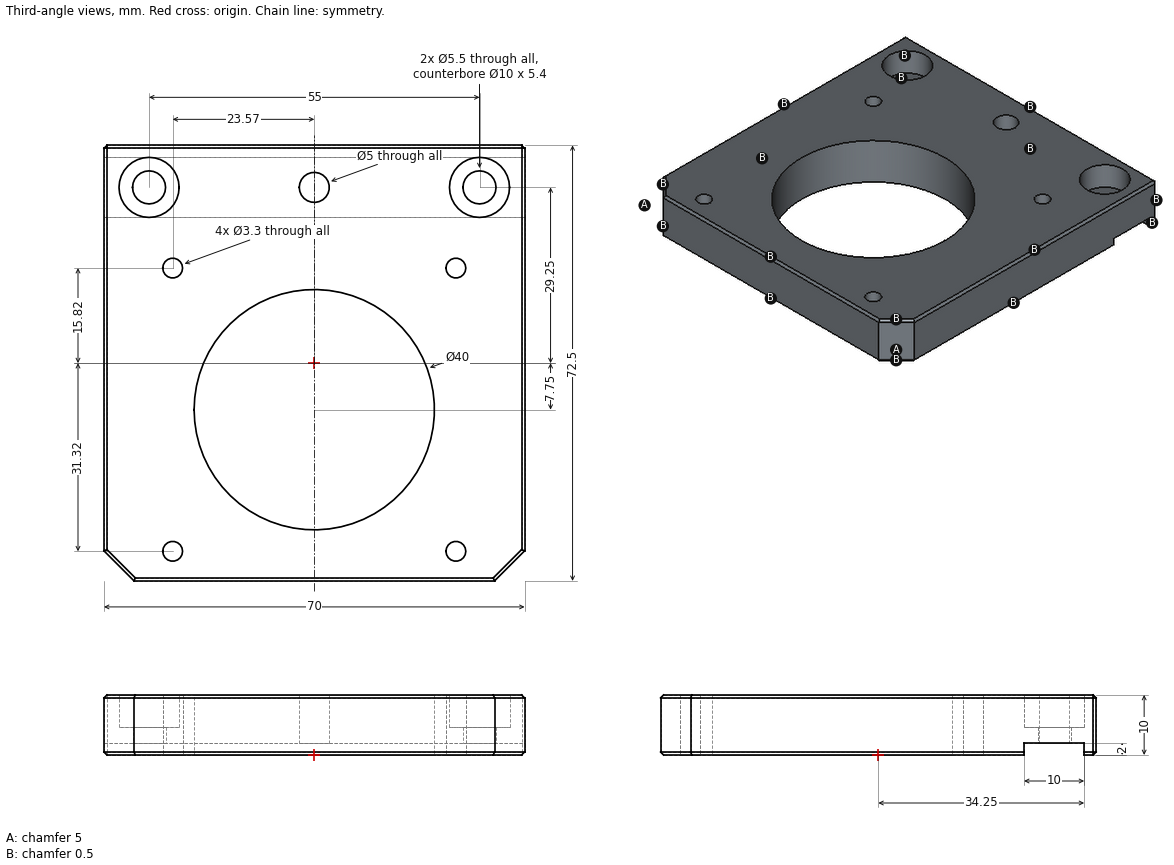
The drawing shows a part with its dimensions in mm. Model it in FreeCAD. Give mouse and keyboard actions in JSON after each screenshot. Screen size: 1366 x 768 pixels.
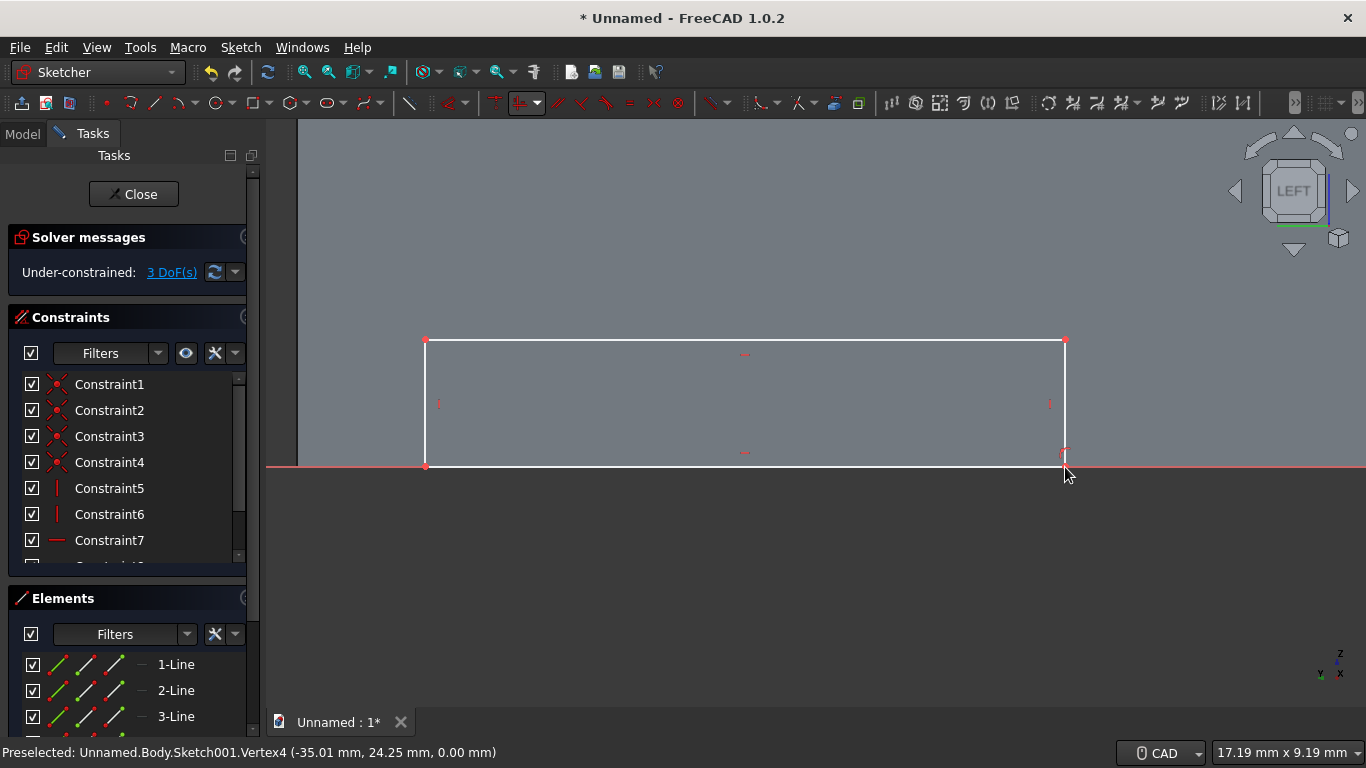
{"action": "left_click", "coordinate": [448, 104]}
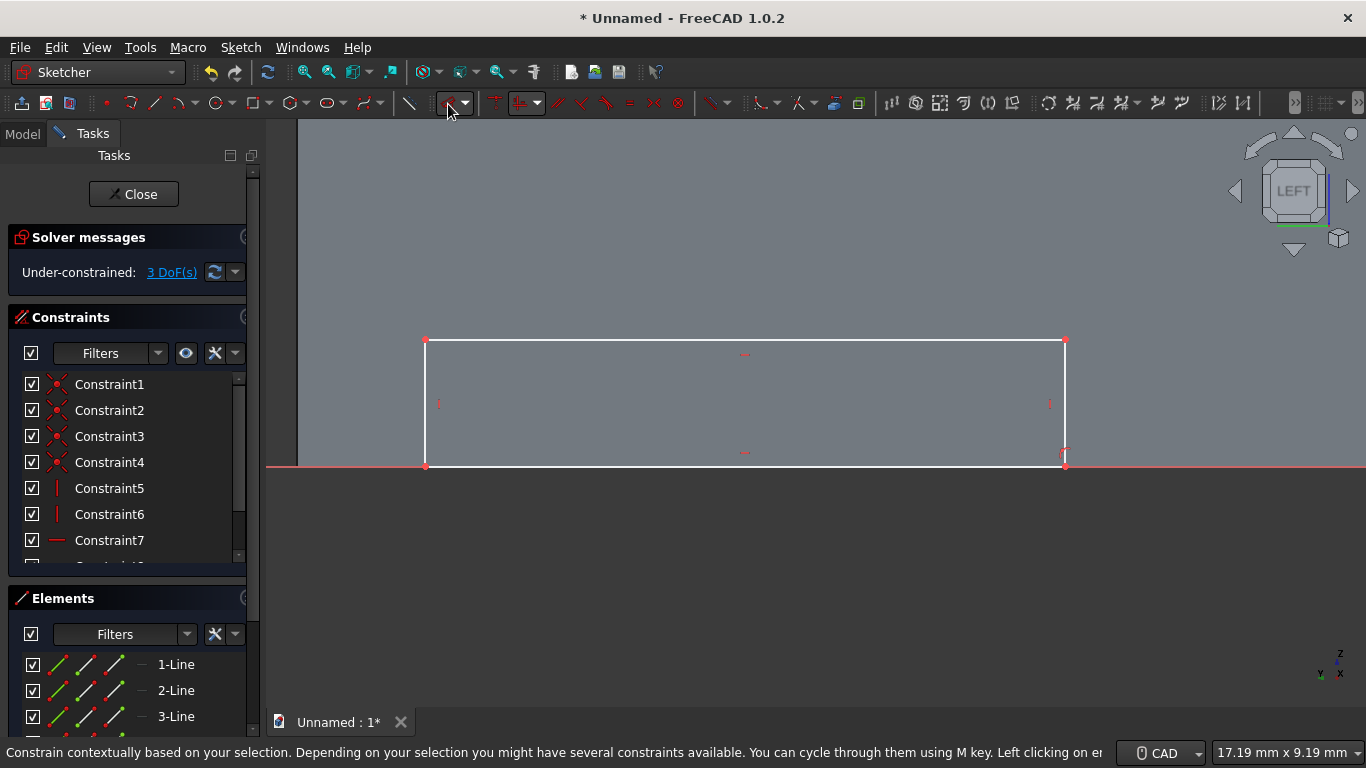
{"action": "left_click", "coordinate": [425, 378]}
{"action": "left_click", "coordinate": [391, 403]}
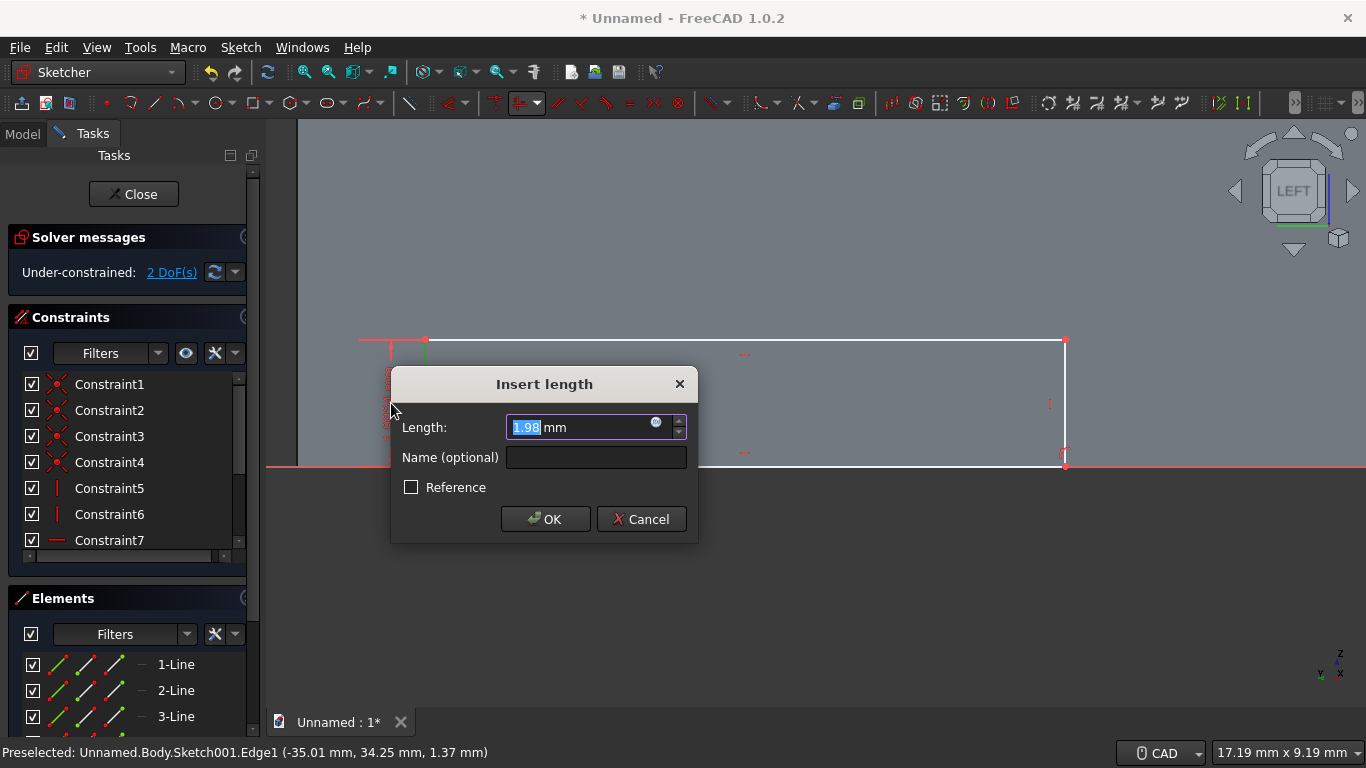
{"action": "type", "text": "2"}
{"action": "key", "text": "Return"}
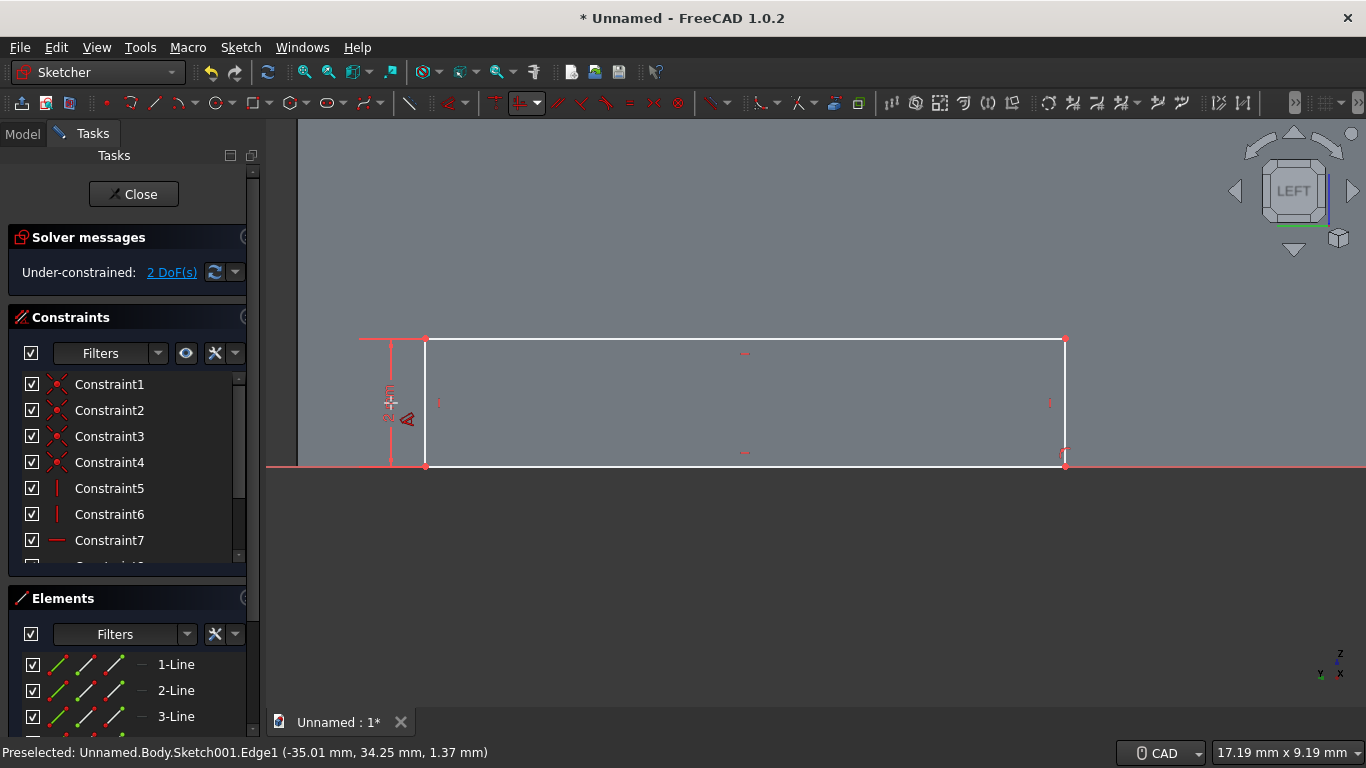
{"action": "left_click", "coordinate": [617, 467]}
{"action": "left_click", "coordinate": [745, 501]}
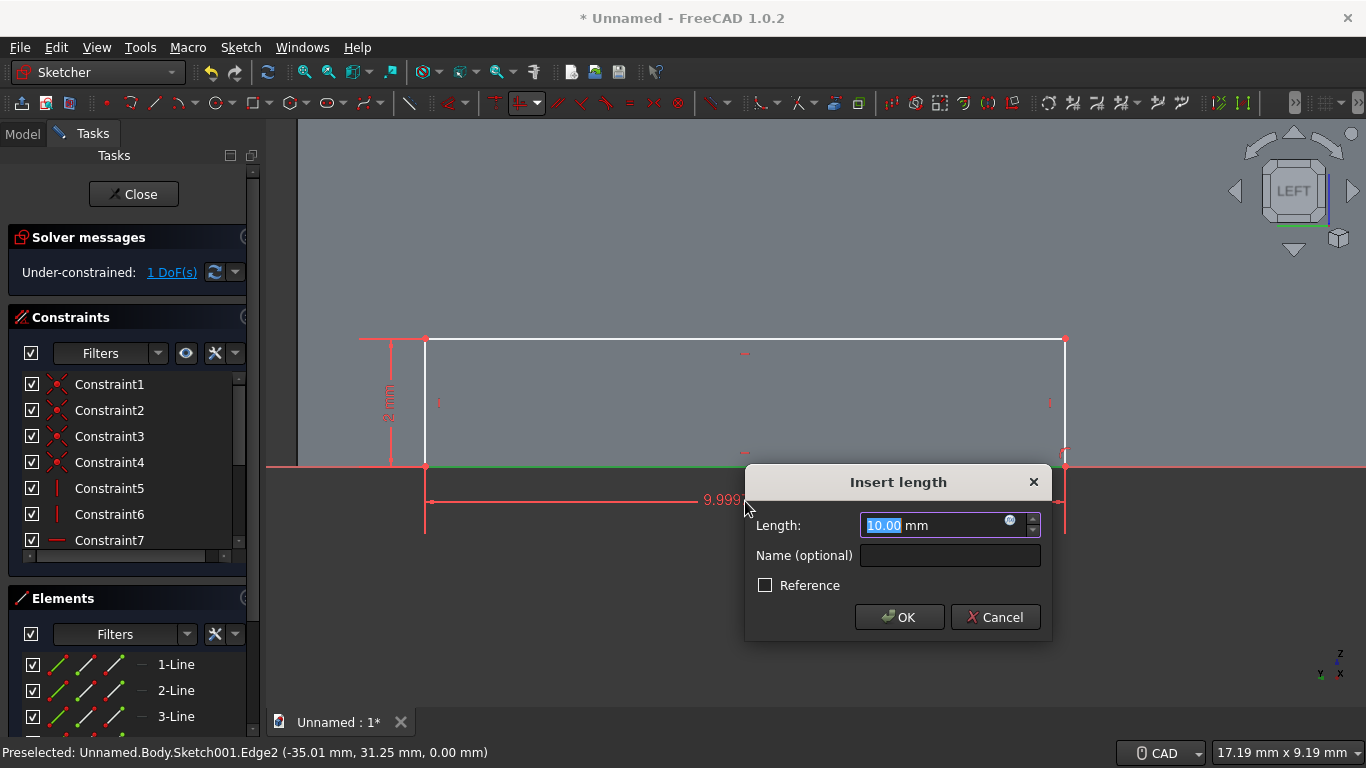
{"action": "type", "text": "10"}
{"action": "key", "text": "Return"}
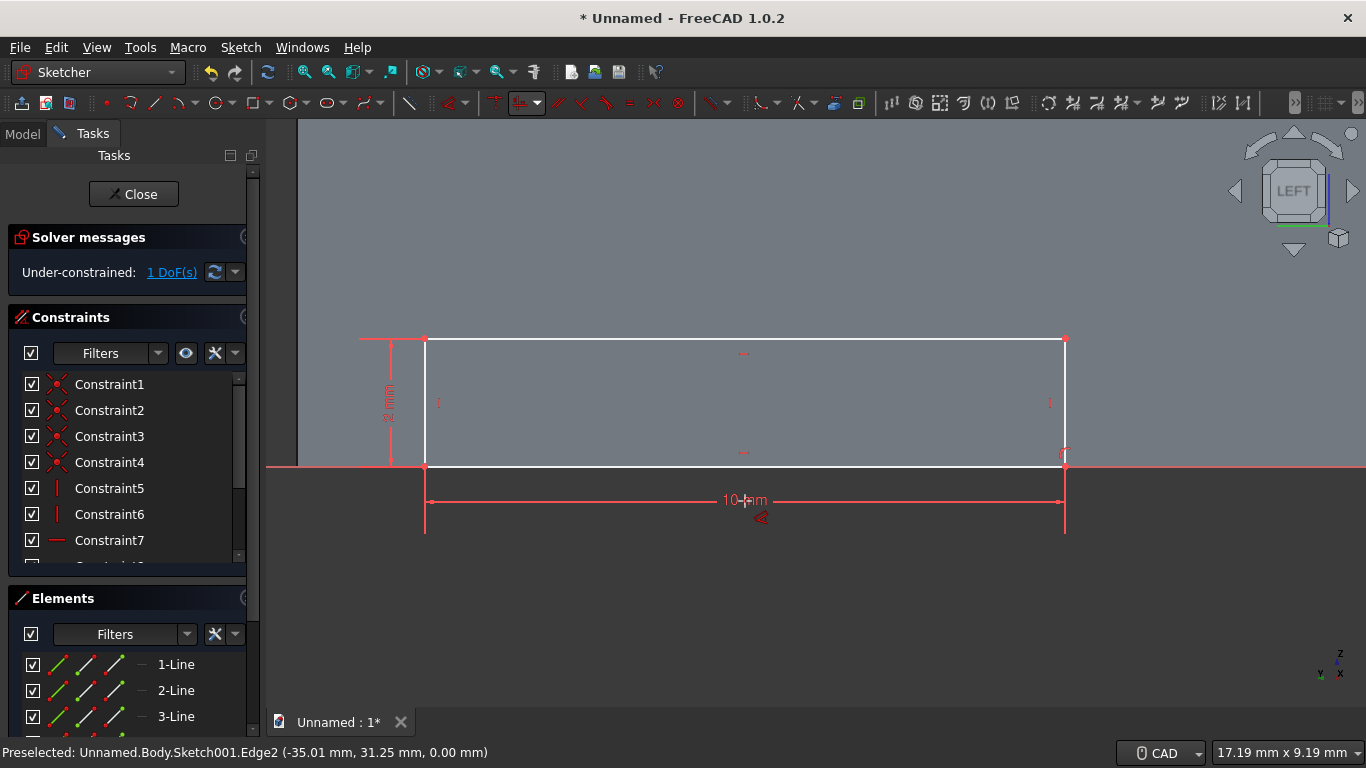
{"action": "left_click", "coordinate": [425, 339]}
{"action": "left_click", "coordinate": [635, 501]}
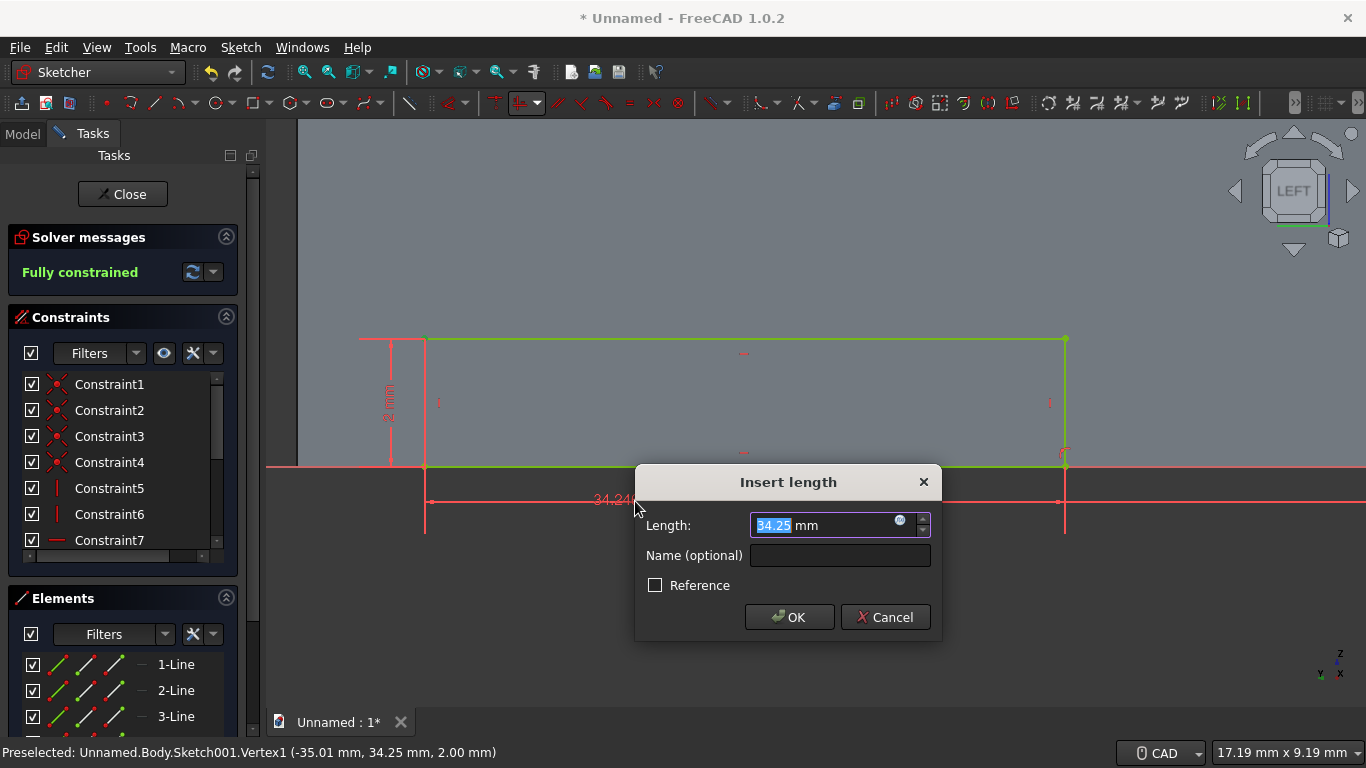
{"action": "type", "text": "34.25"}
{"action": "key", "text": "Return"}
{"action": "key", "text": "Escape"}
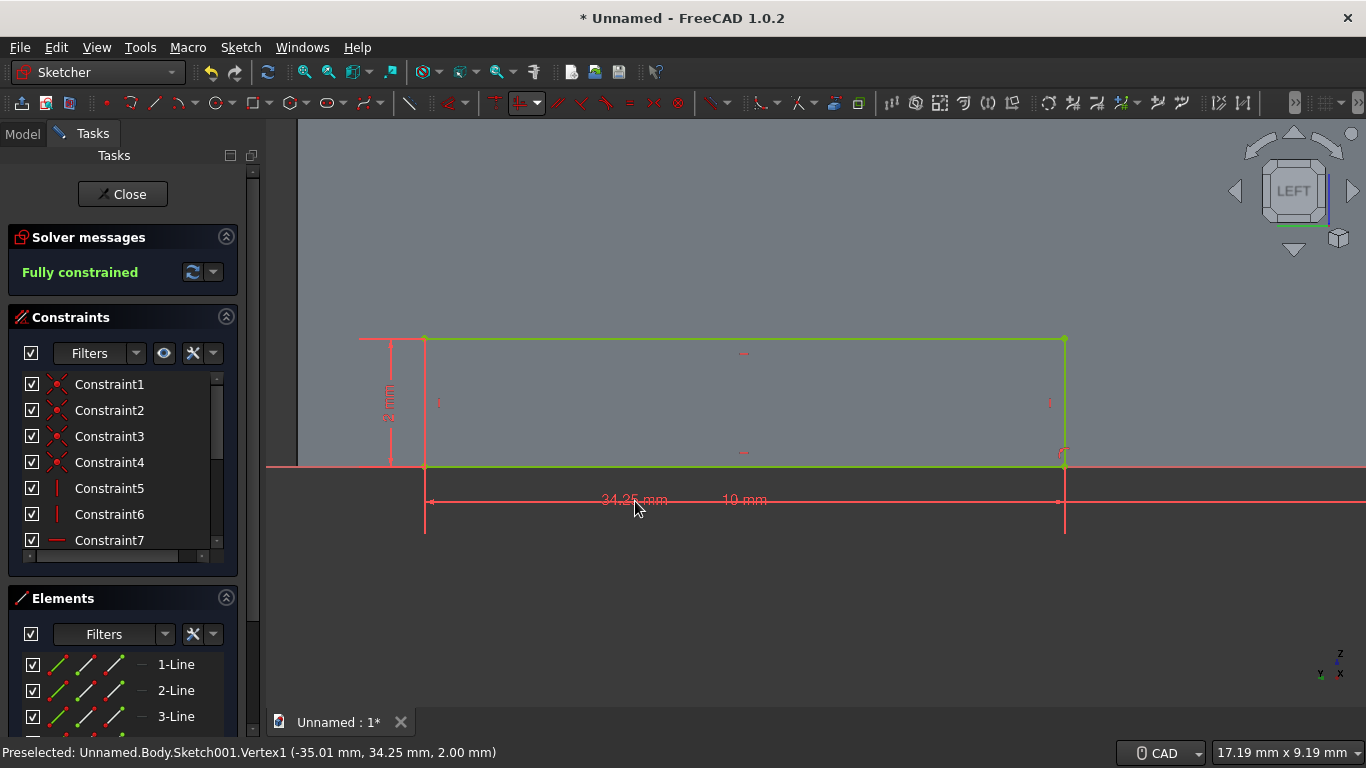
{"action": "left_click", "coordinate": [123, 194]}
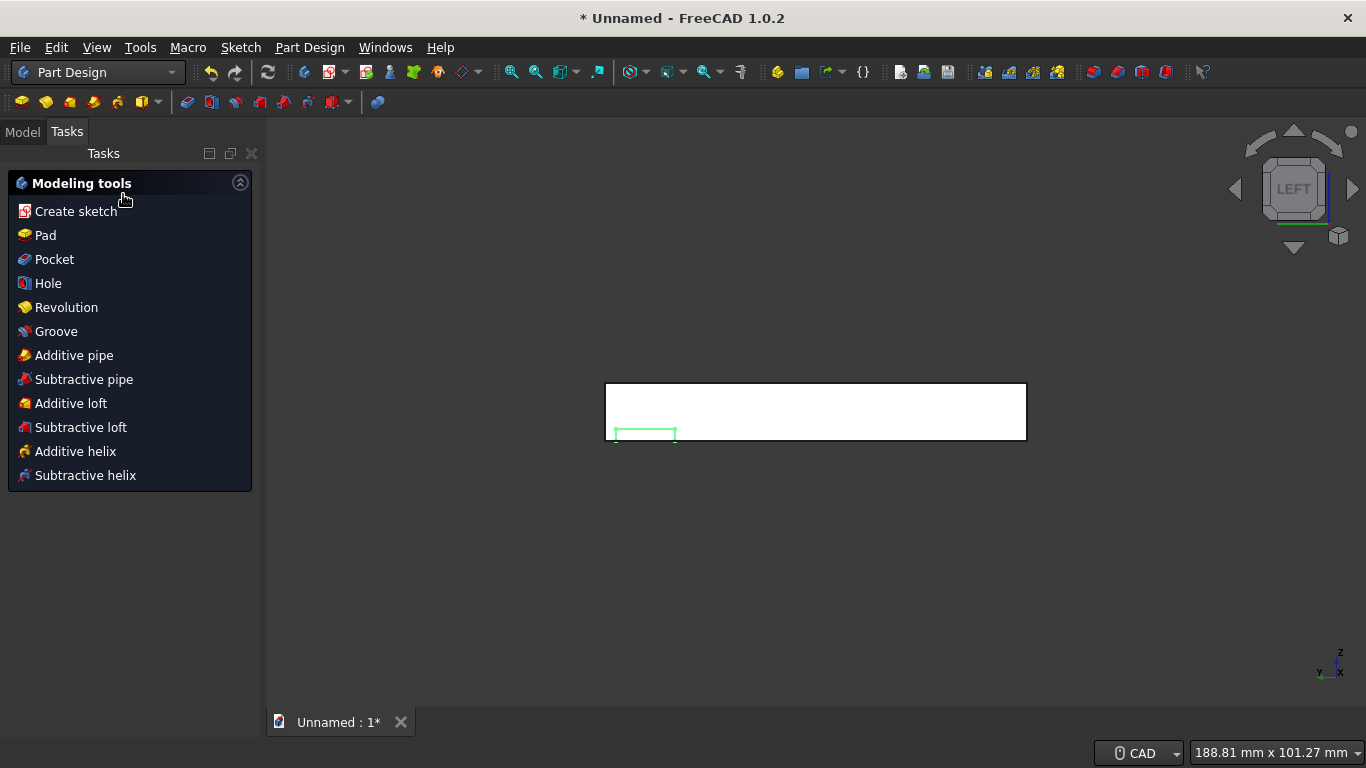
{"action": "left_click", "coordinate": [188, 102]}